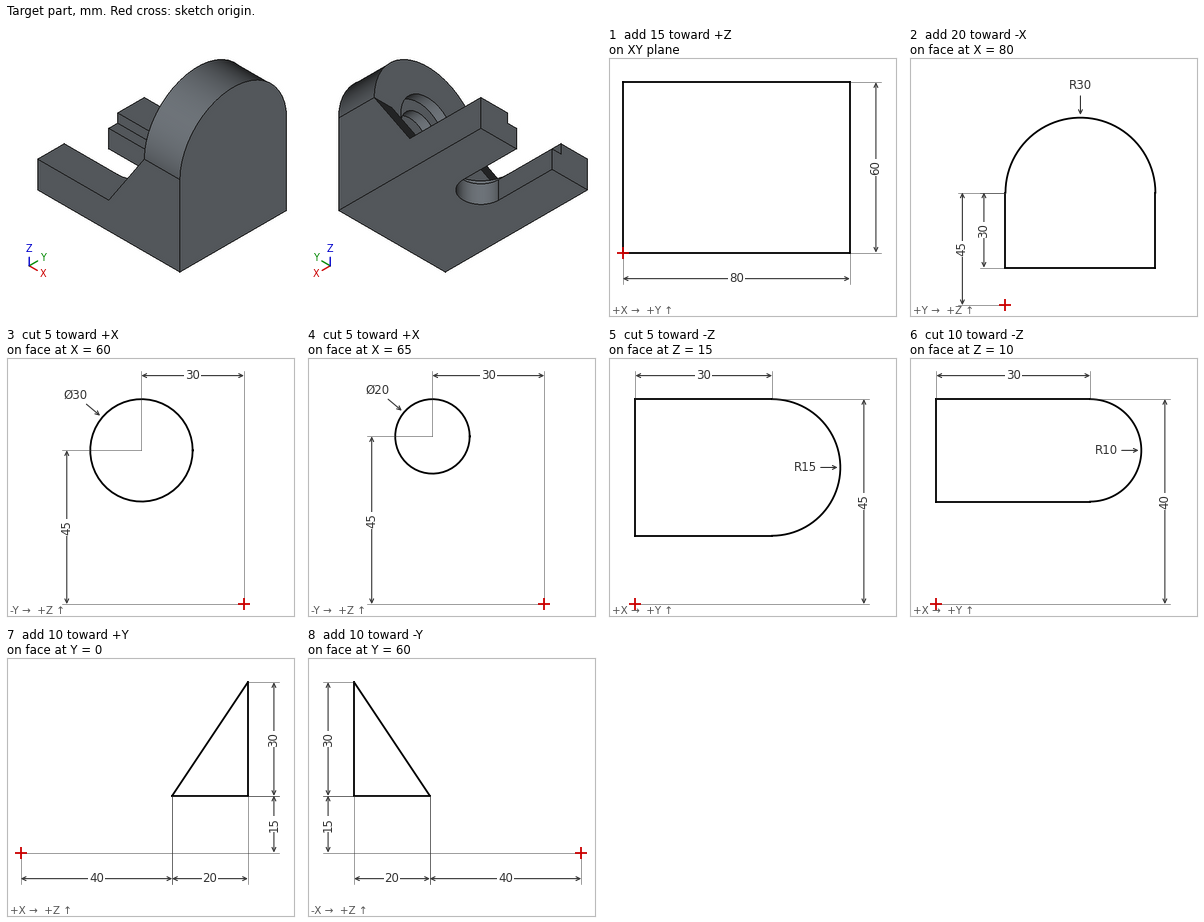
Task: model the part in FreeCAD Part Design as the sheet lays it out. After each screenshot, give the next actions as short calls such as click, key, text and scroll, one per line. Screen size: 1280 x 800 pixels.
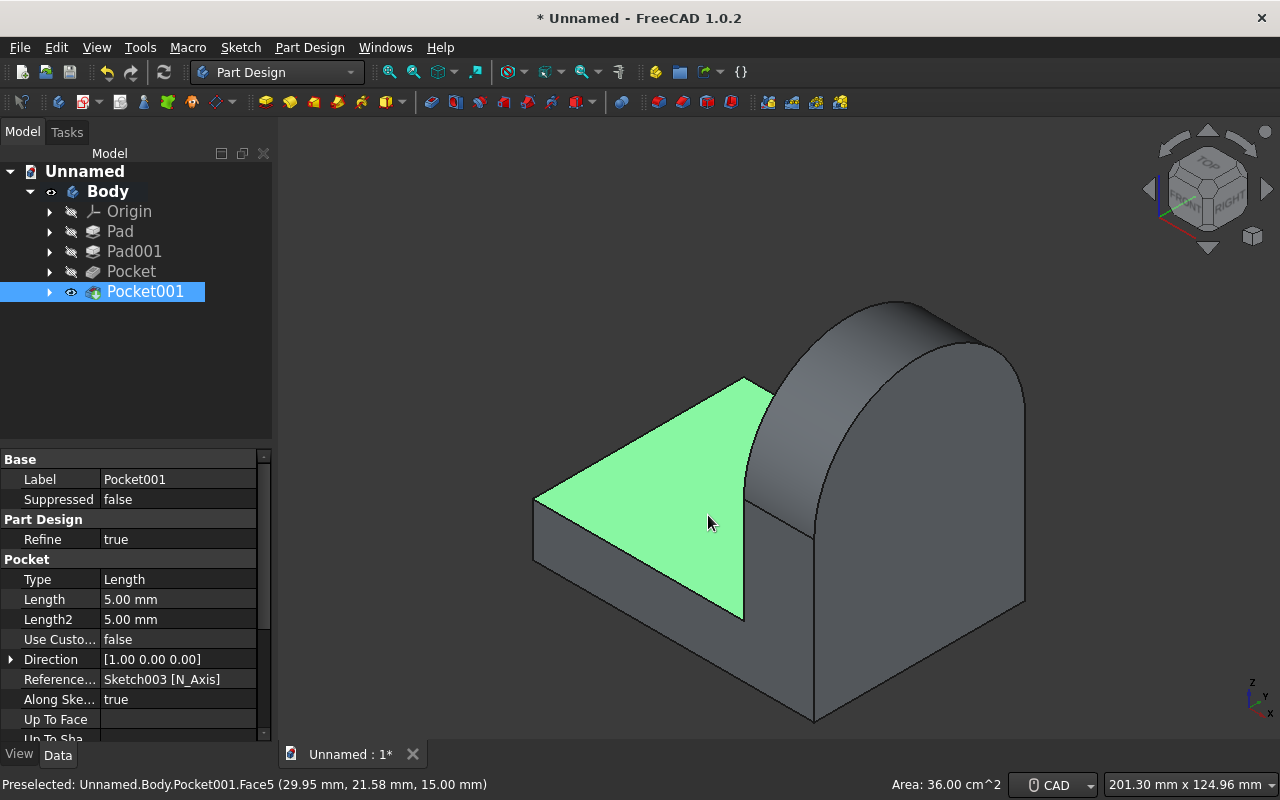
click(84, 102)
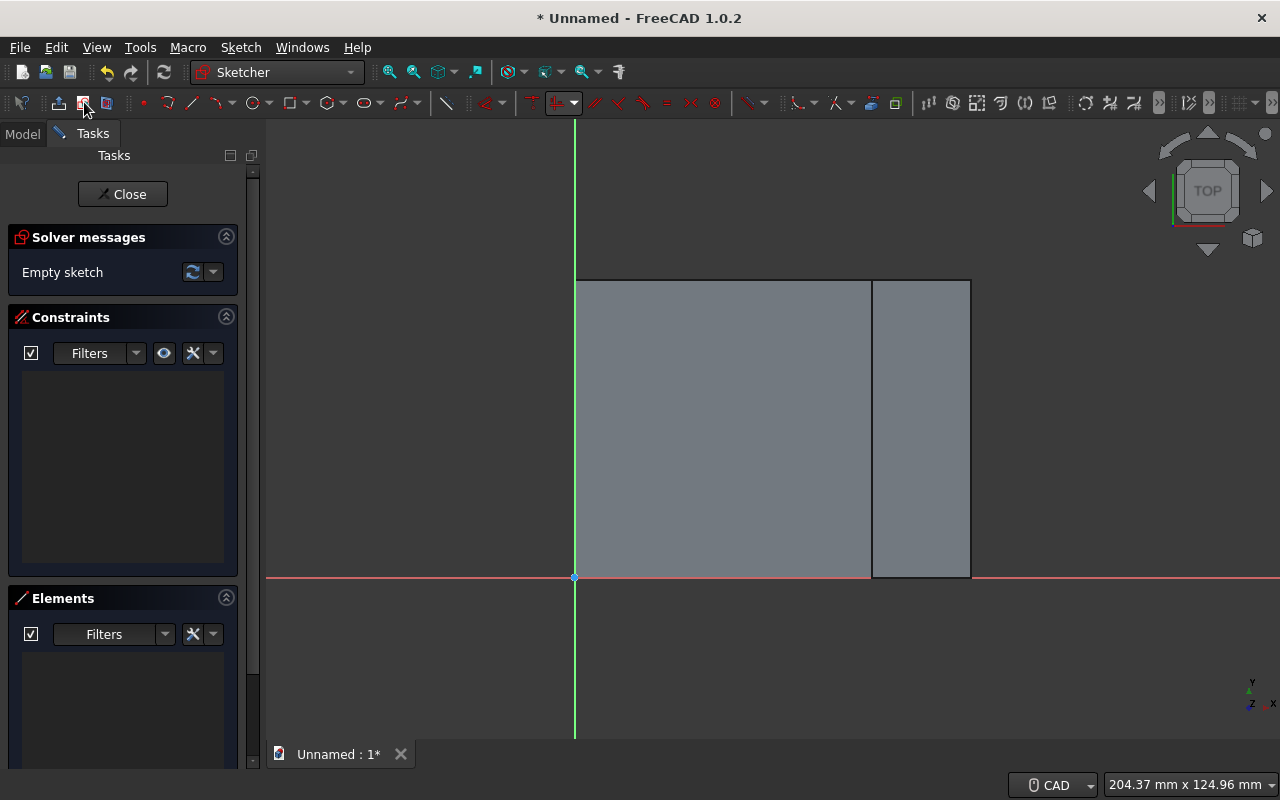
scroll(664, 511, up, 3)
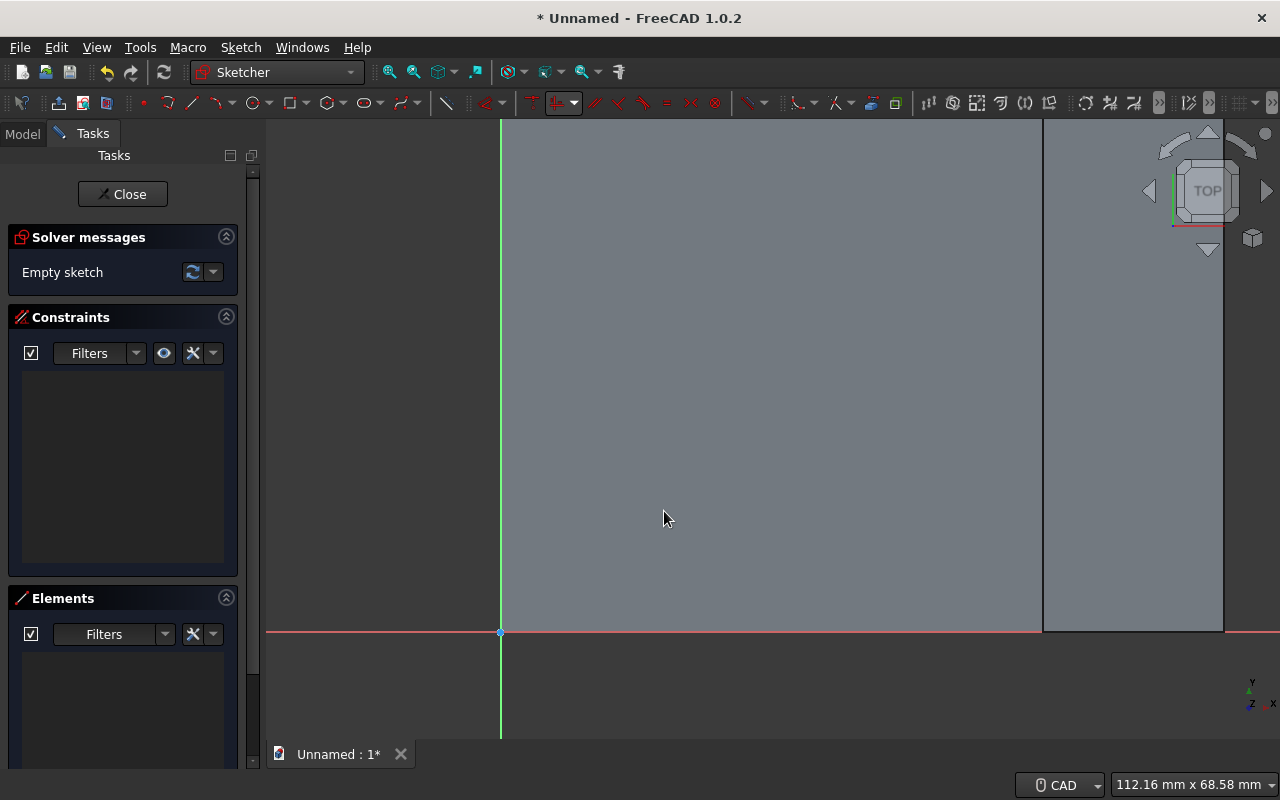
click(168, 104)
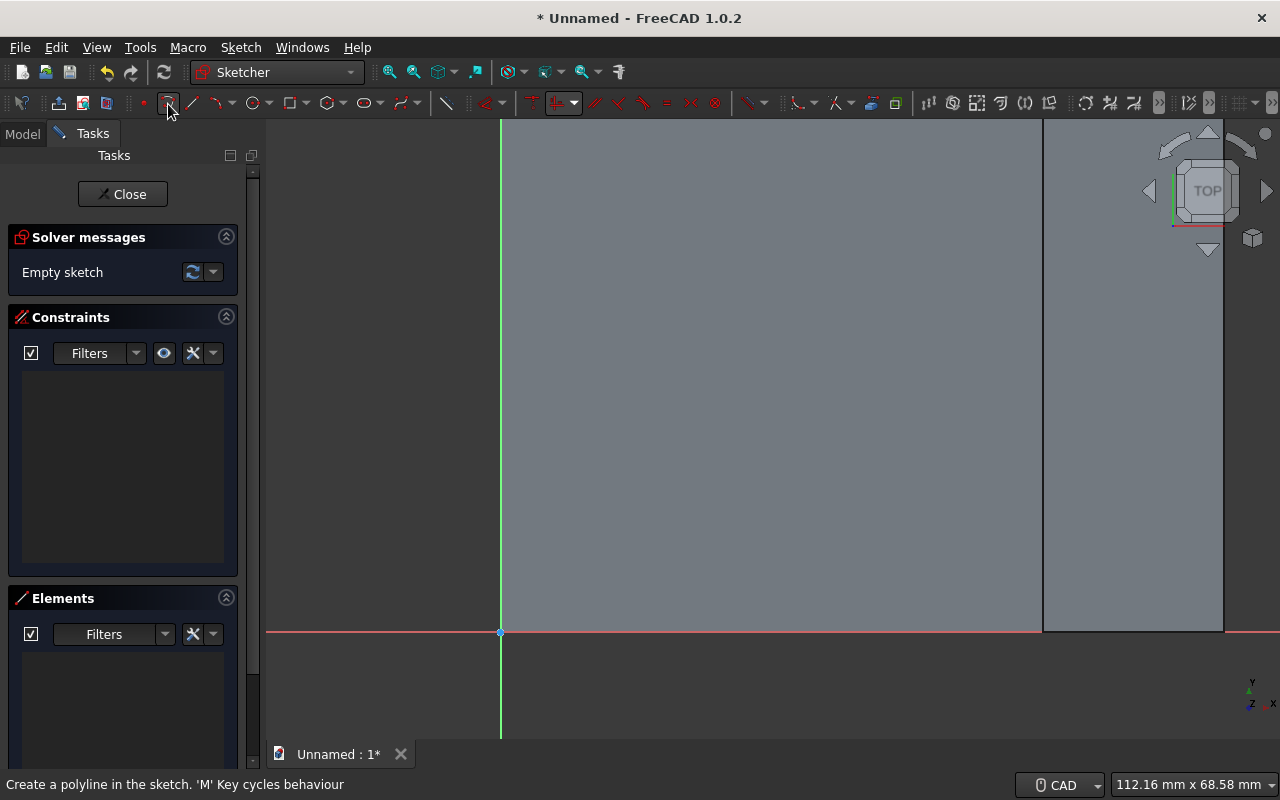
click(772, 225)
click(501, 225)
click(510, 497)
click(772, 497)
right_click(772, 497)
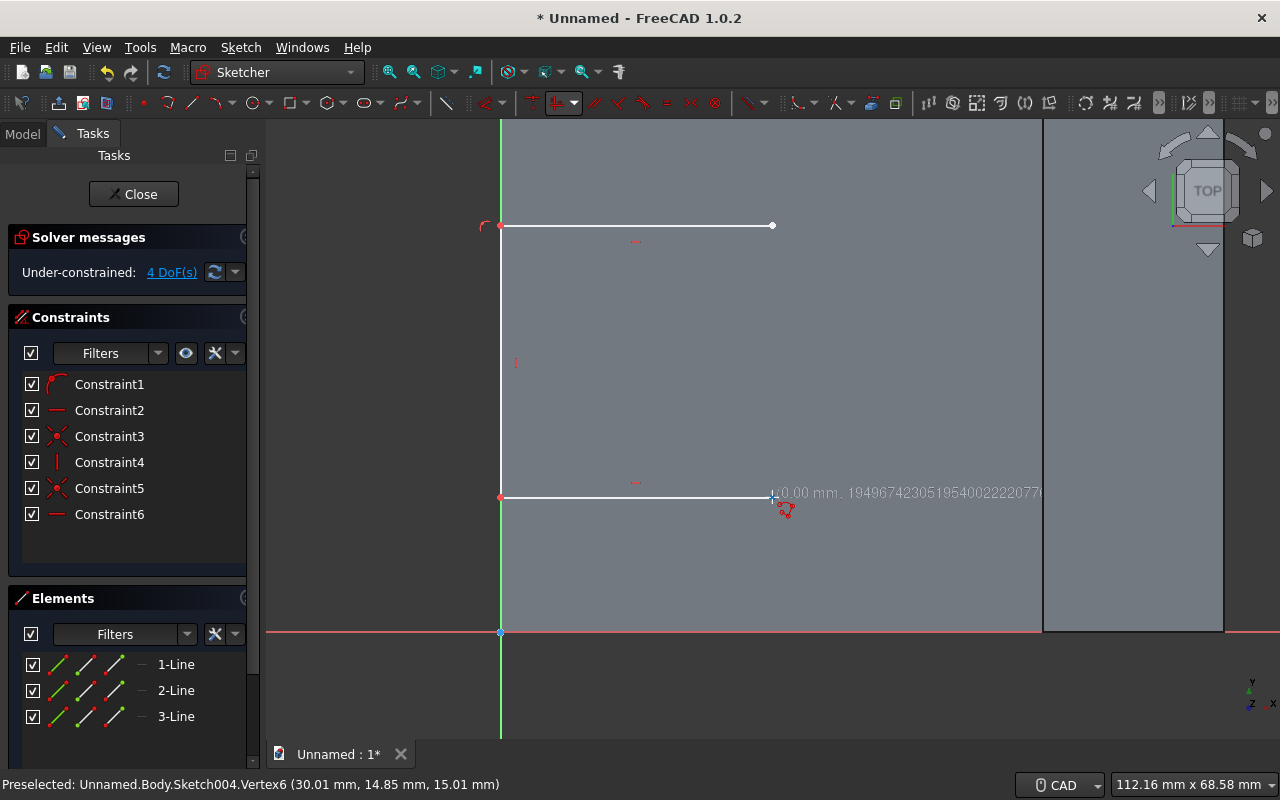
click(216, 104)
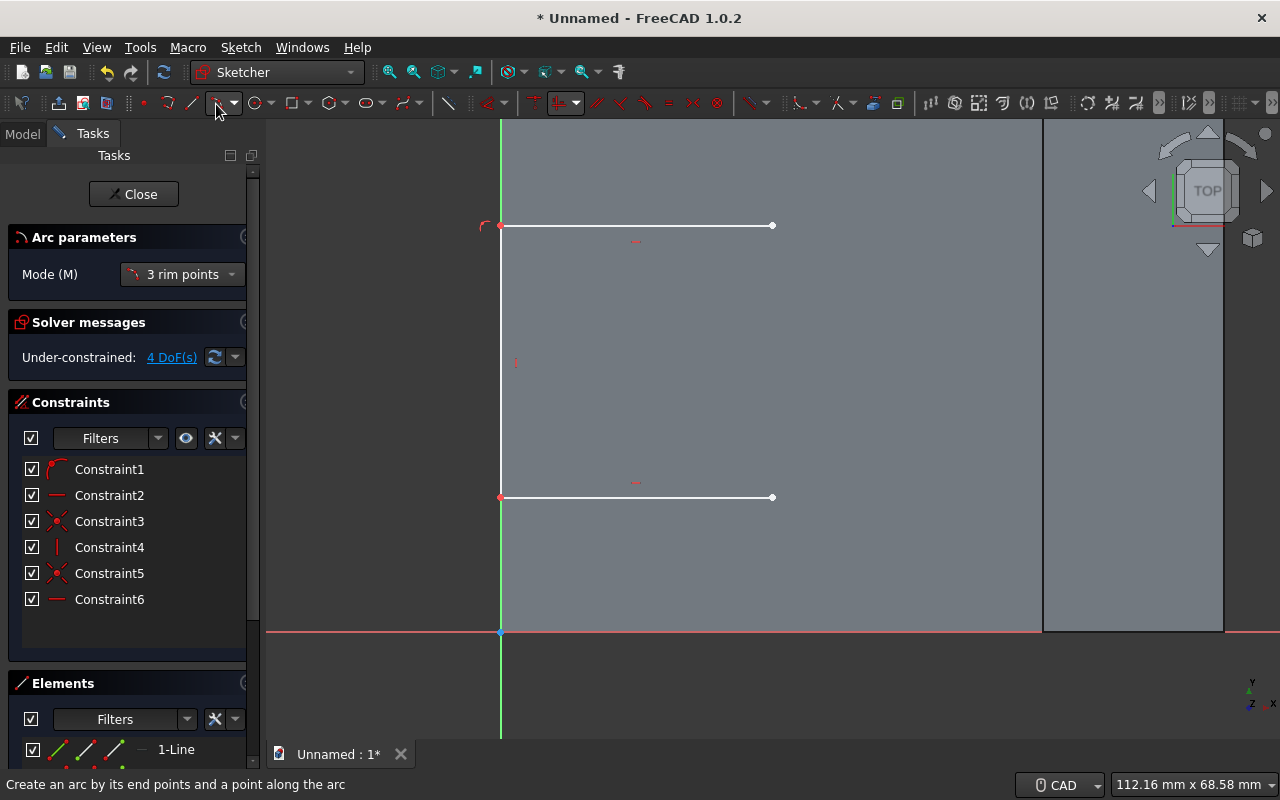
click(772, 498)
click(772, 226)
click(907, 361)
key(Escape)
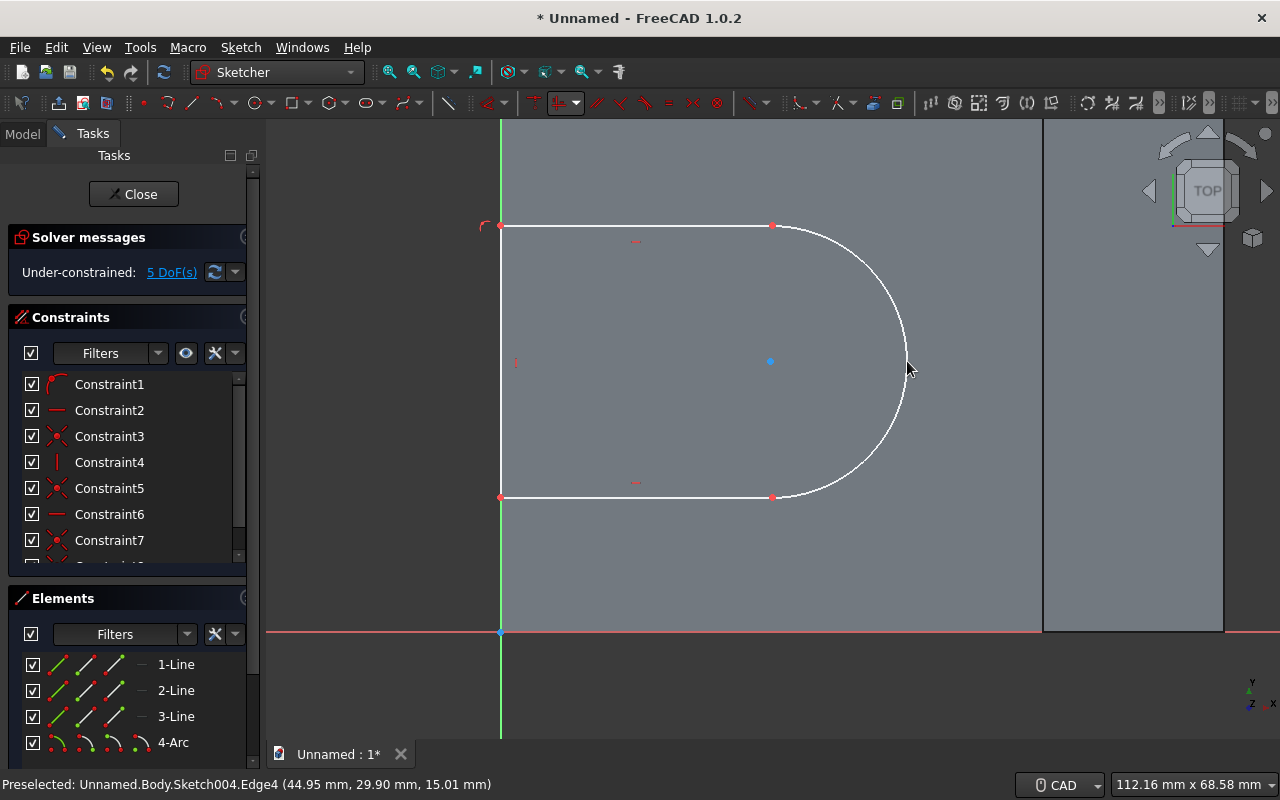
click(691, 226)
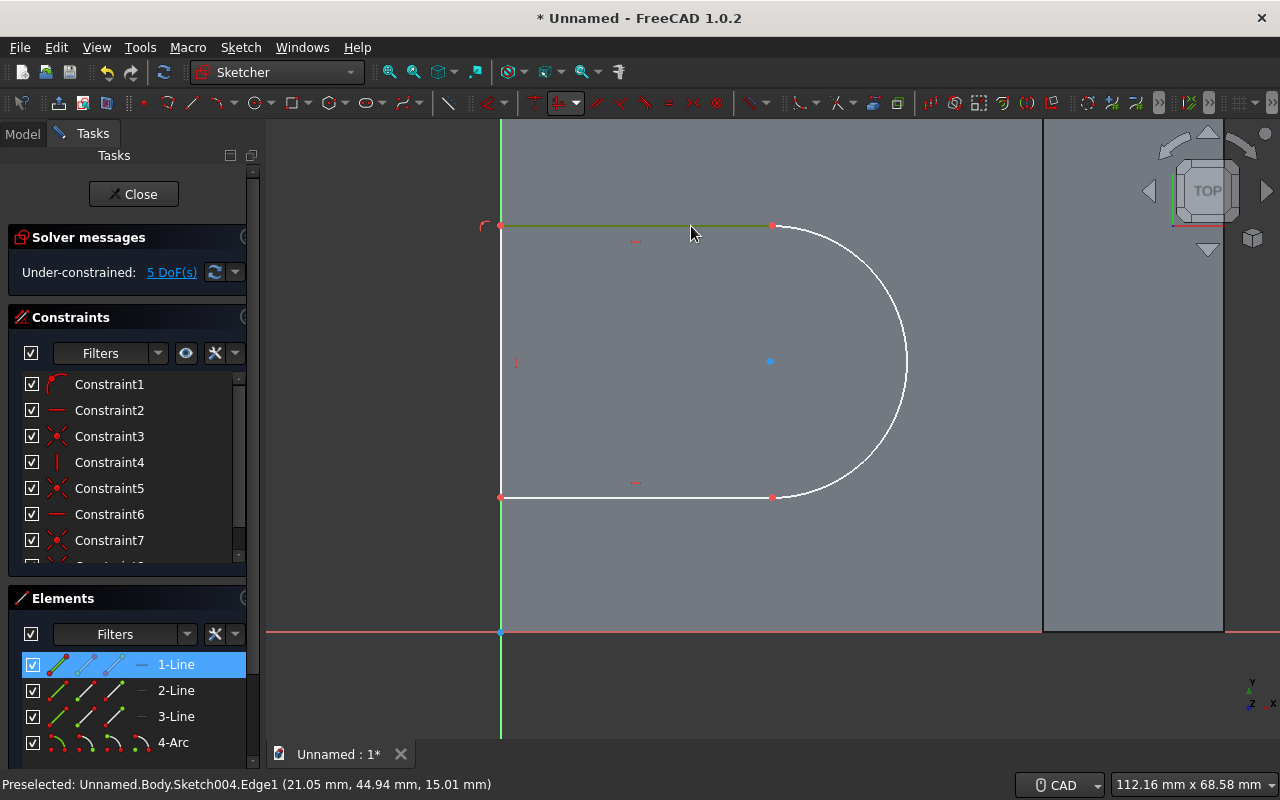
click(881, 442)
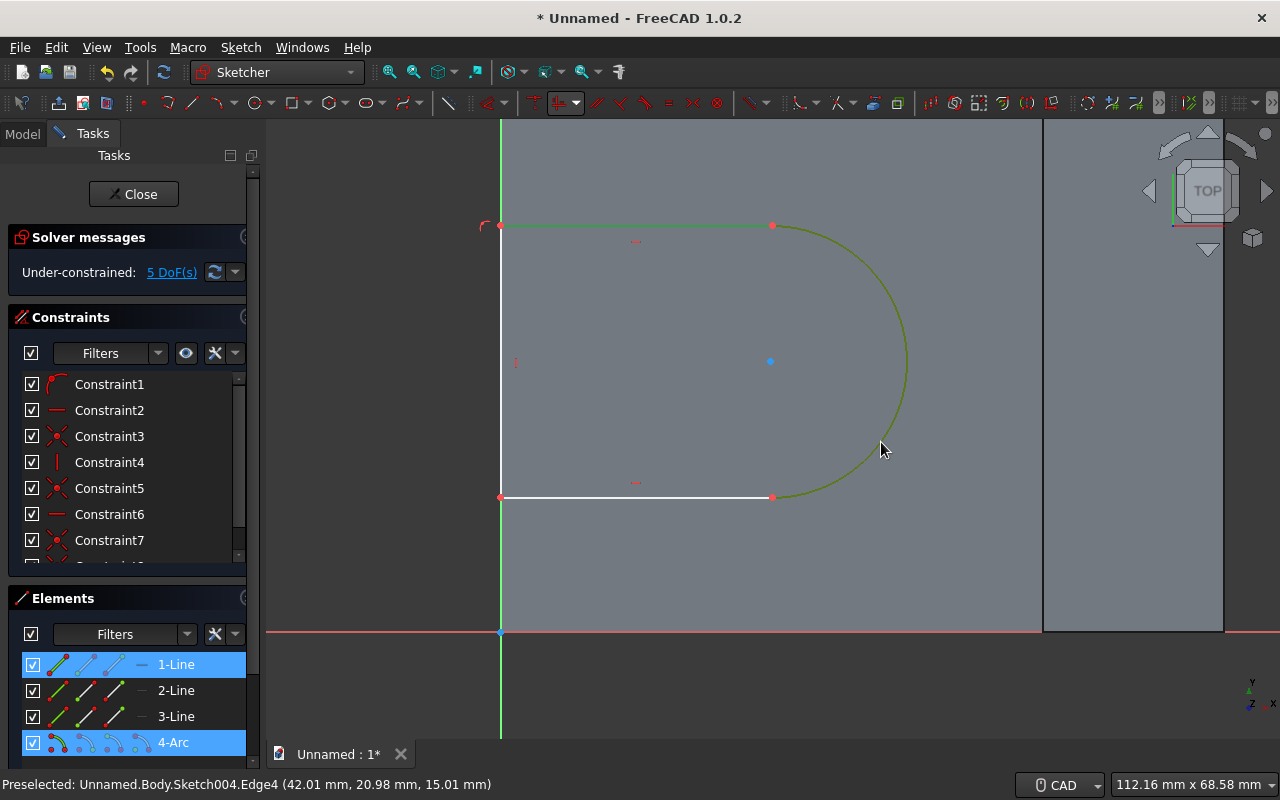
click(646, 104)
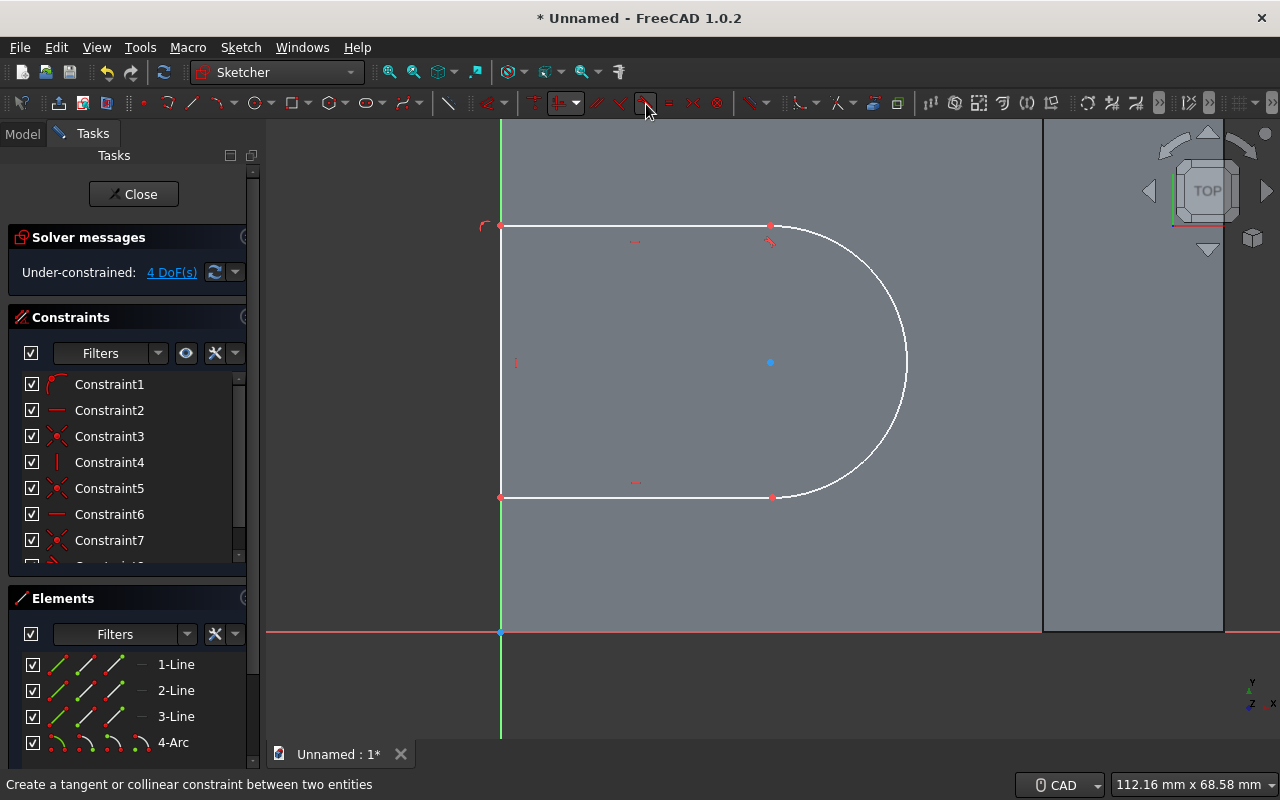
click(582, 498)